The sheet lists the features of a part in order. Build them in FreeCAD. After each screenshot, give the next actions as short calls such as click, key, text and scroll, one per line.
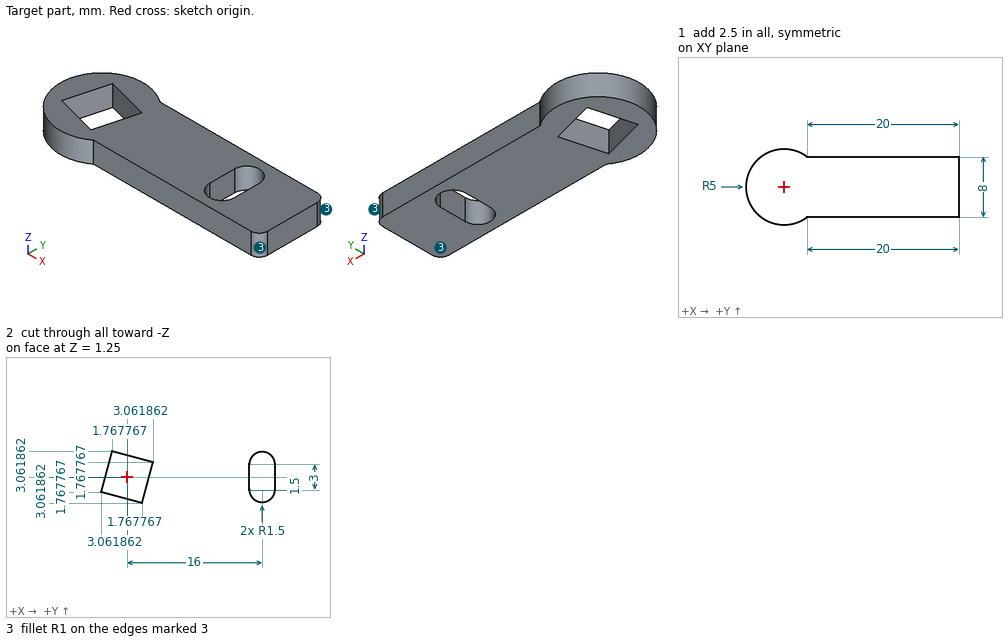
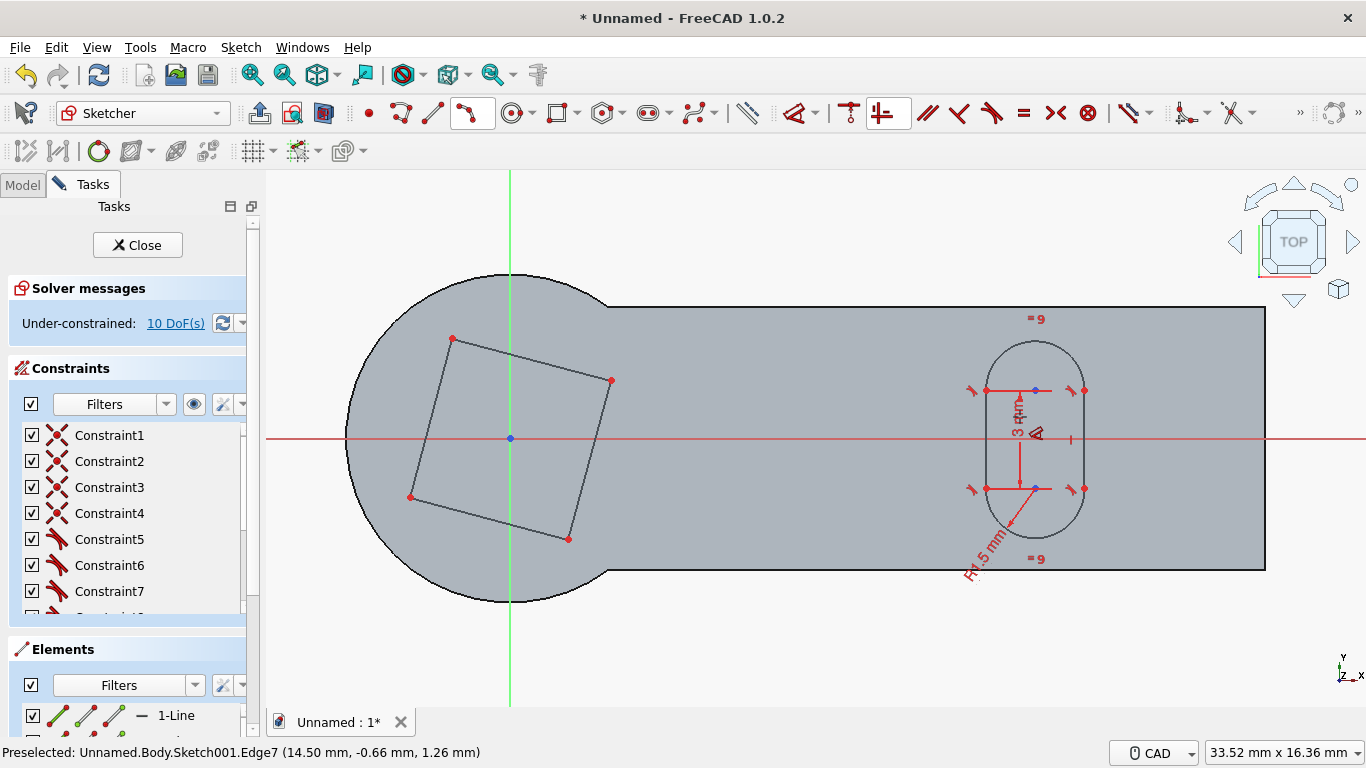
click(1035, 489)
click(773, 523)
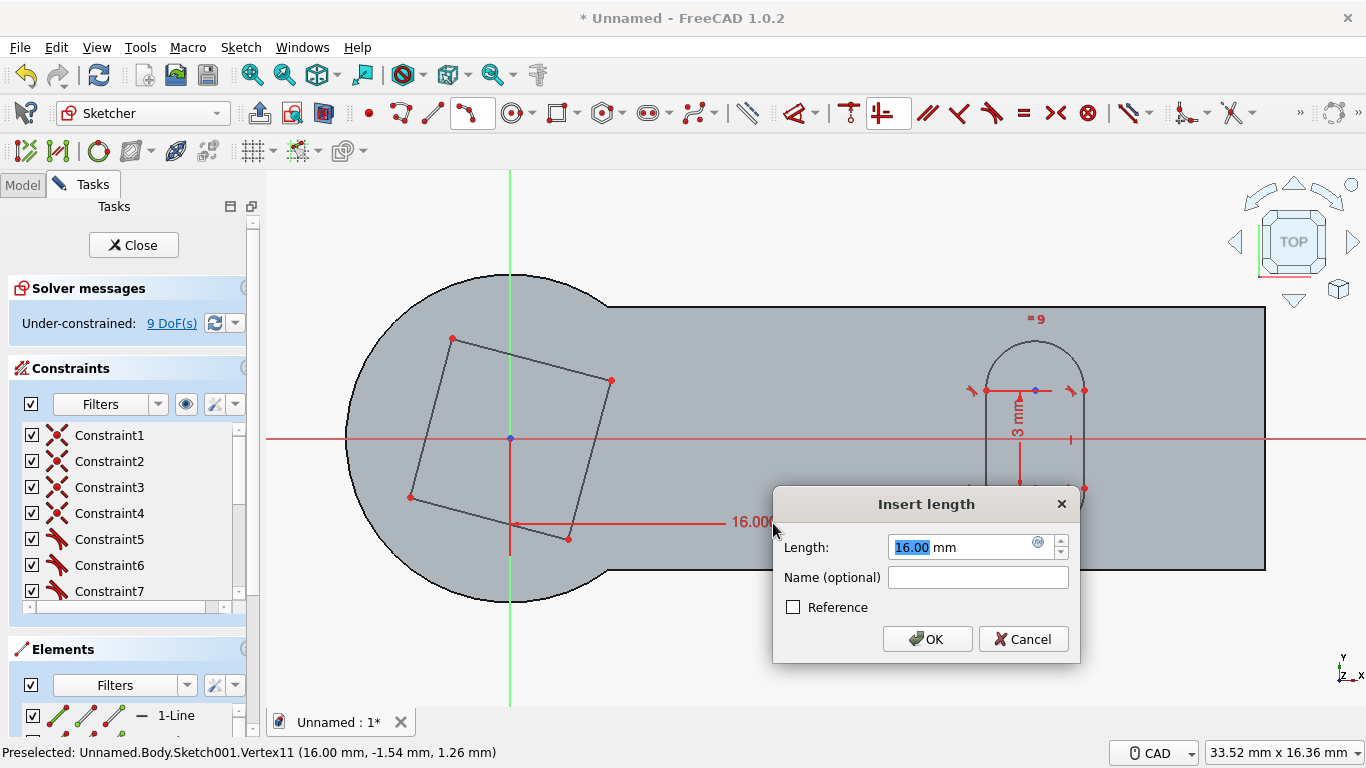
text(16)
key(Return)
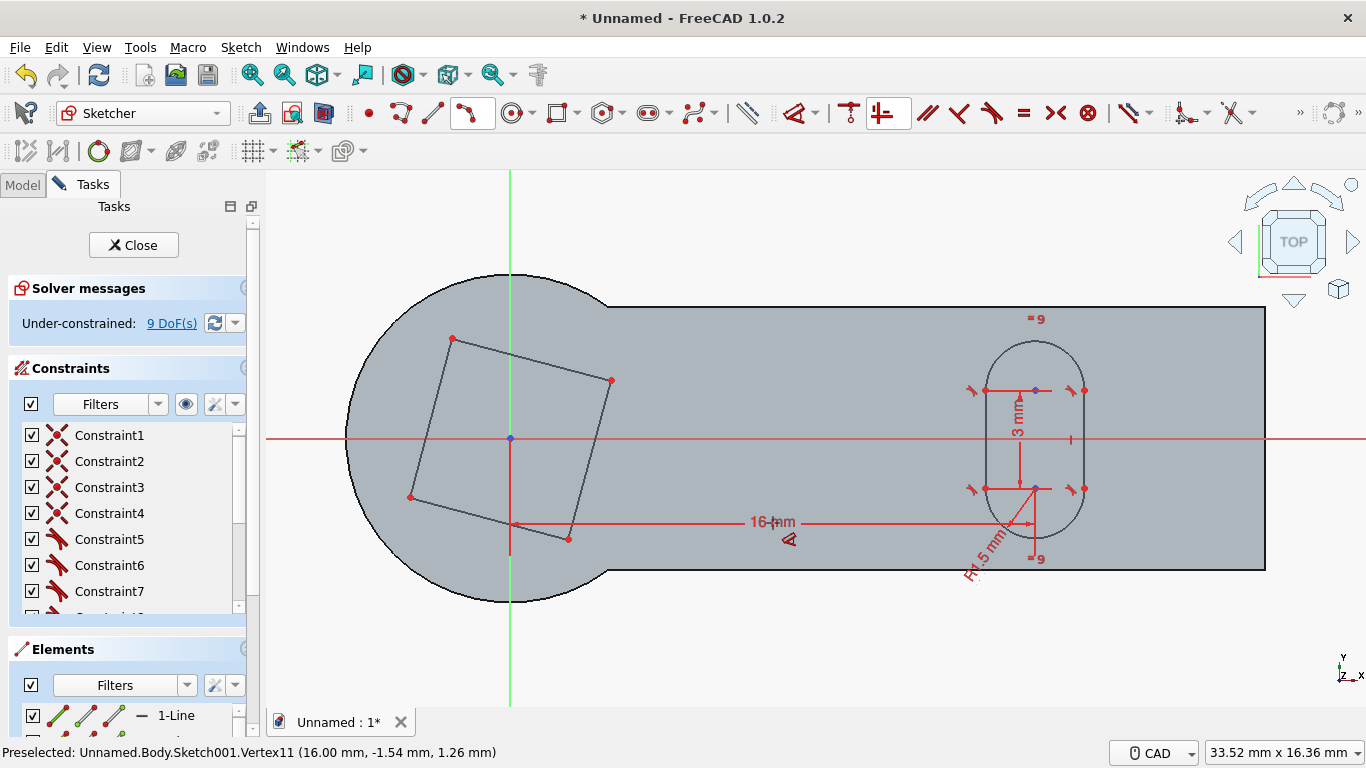
click(986, 489)
click(1020, 464)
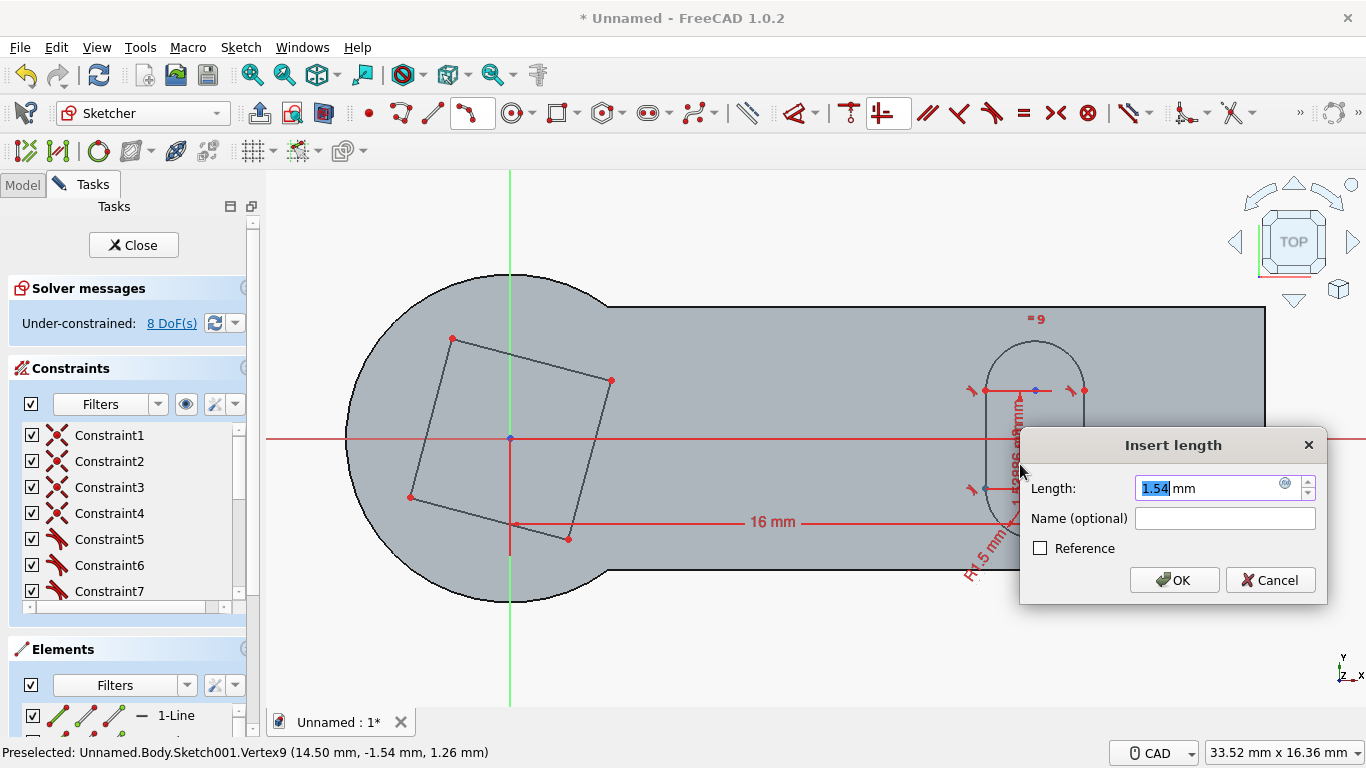
text(1.5)
key(Return)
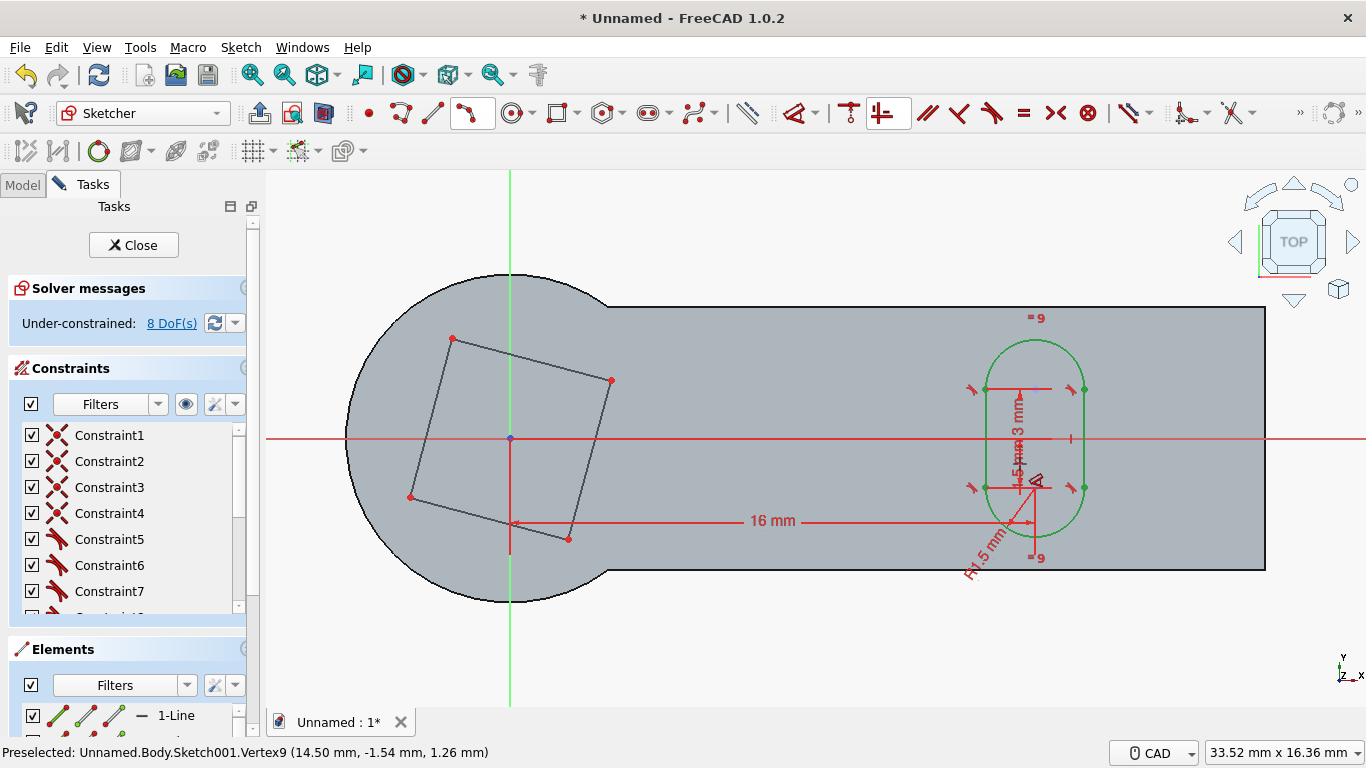
click(568, 540)
click(539, 574)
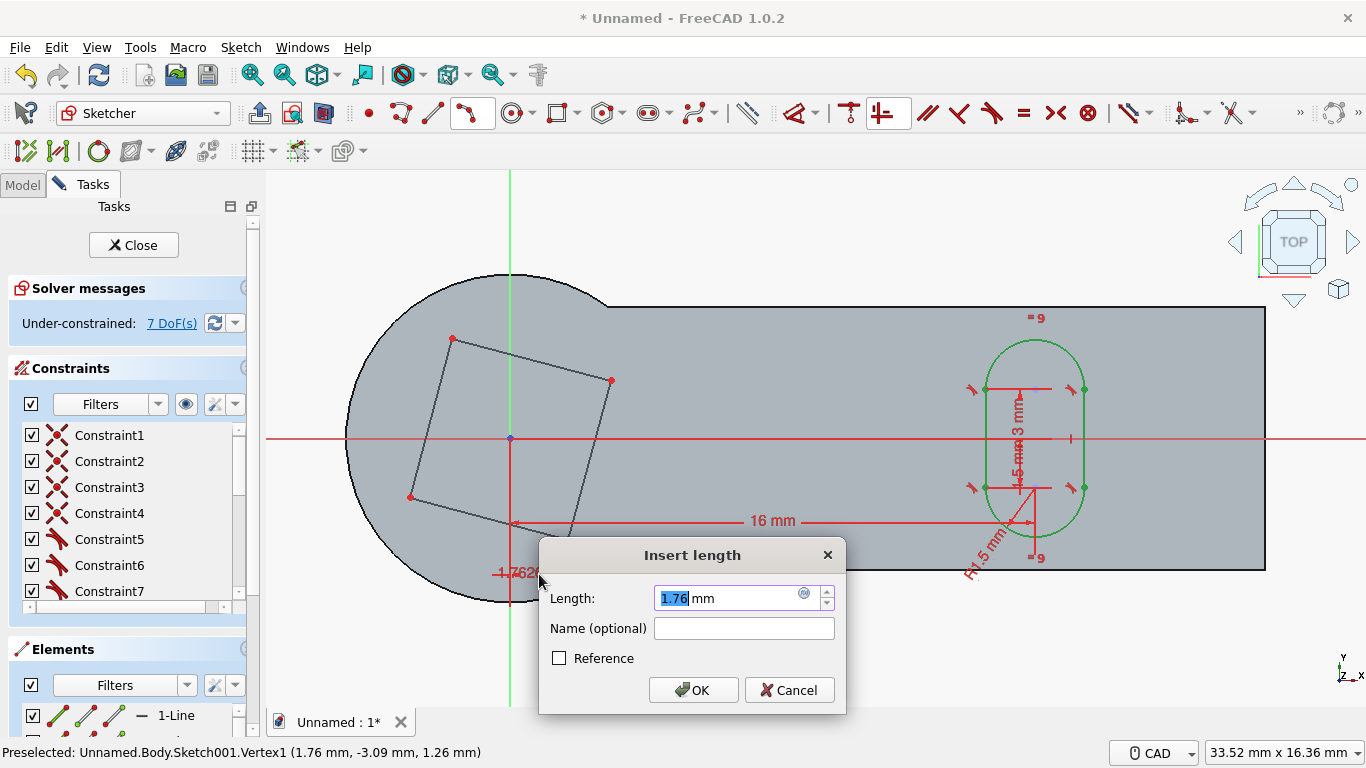
text(1.767767)
key(Return)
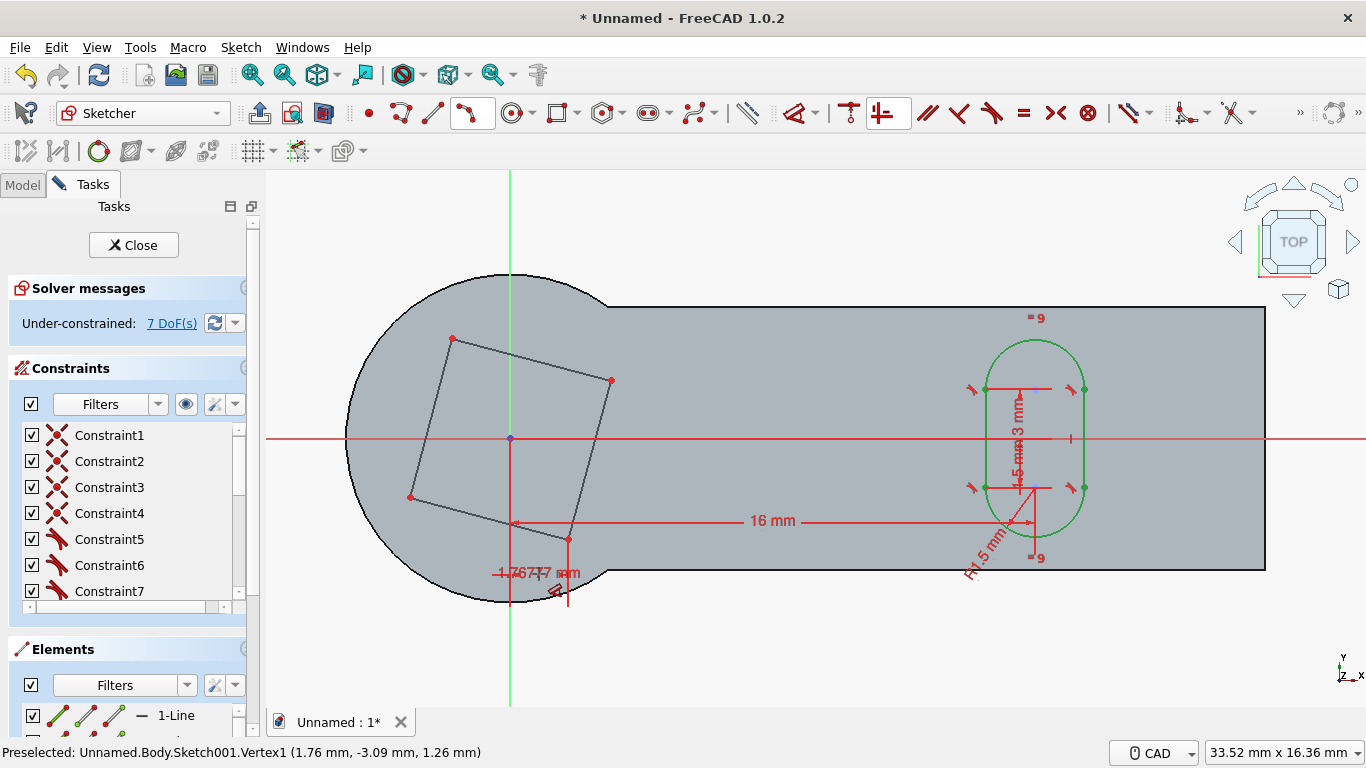
click(568, 540)
click(476, 489)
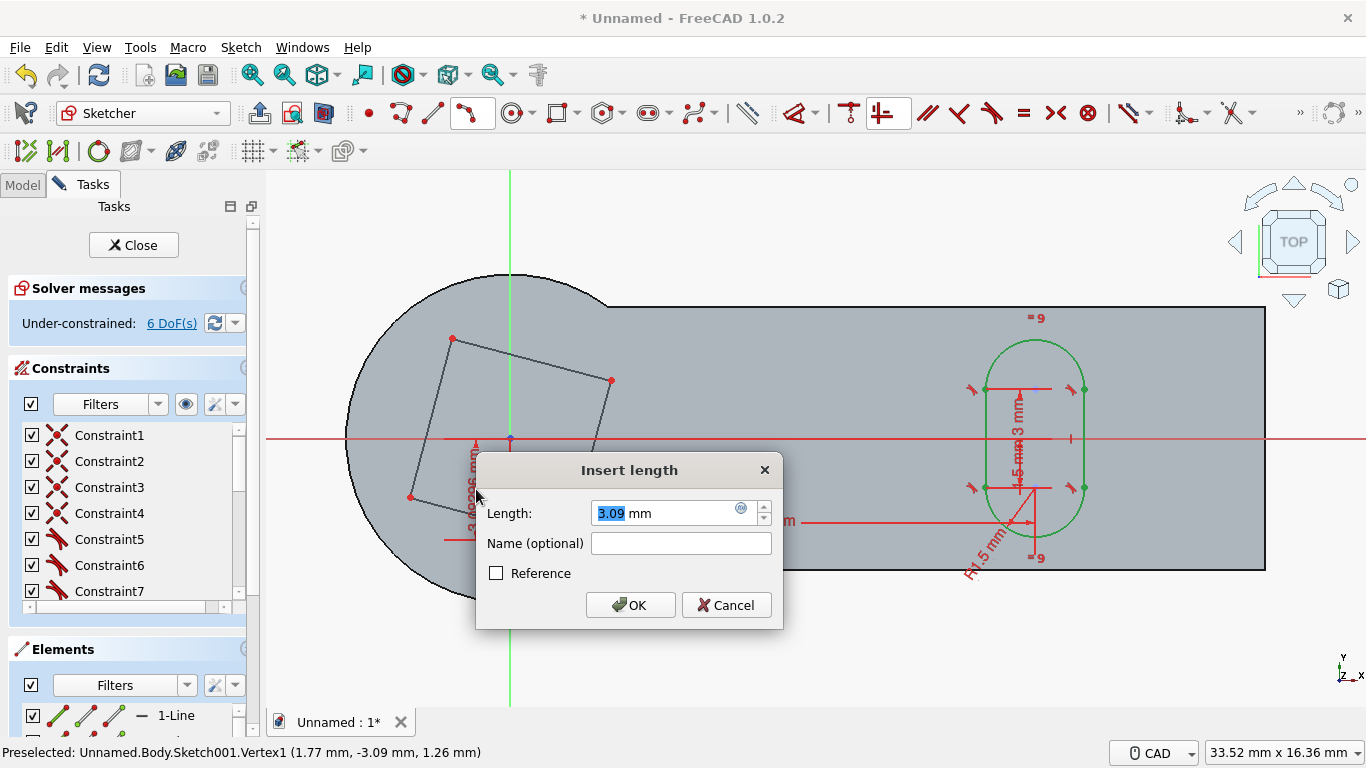
text(3.061862)
key(Return)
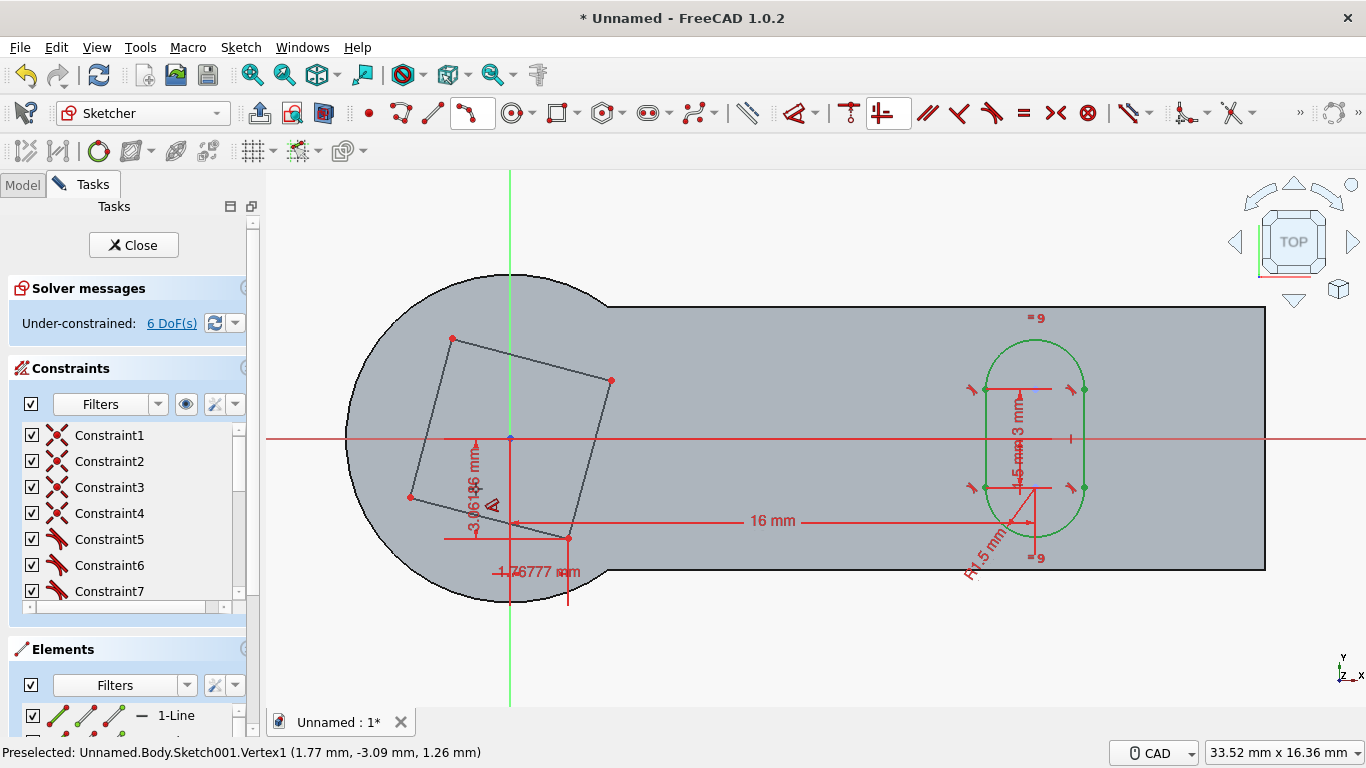
click(611, 381)
click(561, 347)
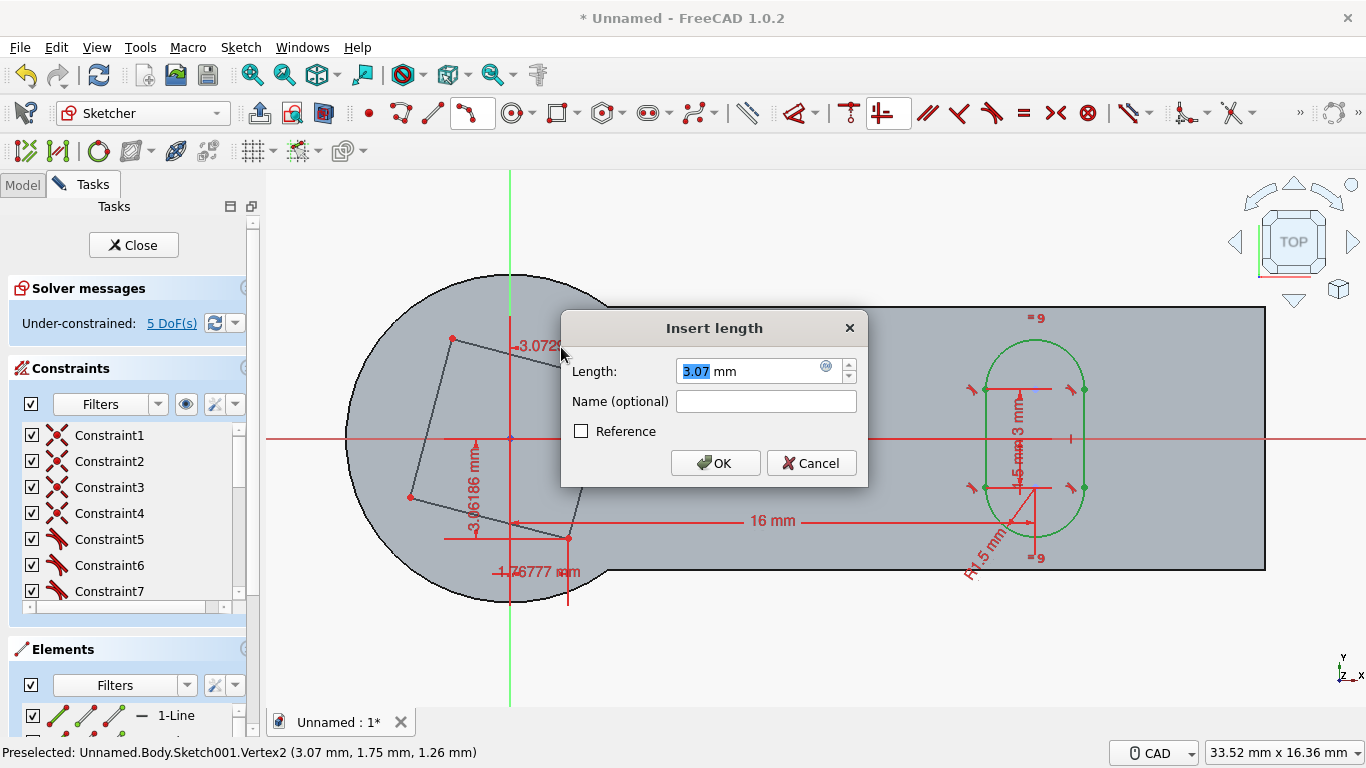
text(3.061862)
key(Return)